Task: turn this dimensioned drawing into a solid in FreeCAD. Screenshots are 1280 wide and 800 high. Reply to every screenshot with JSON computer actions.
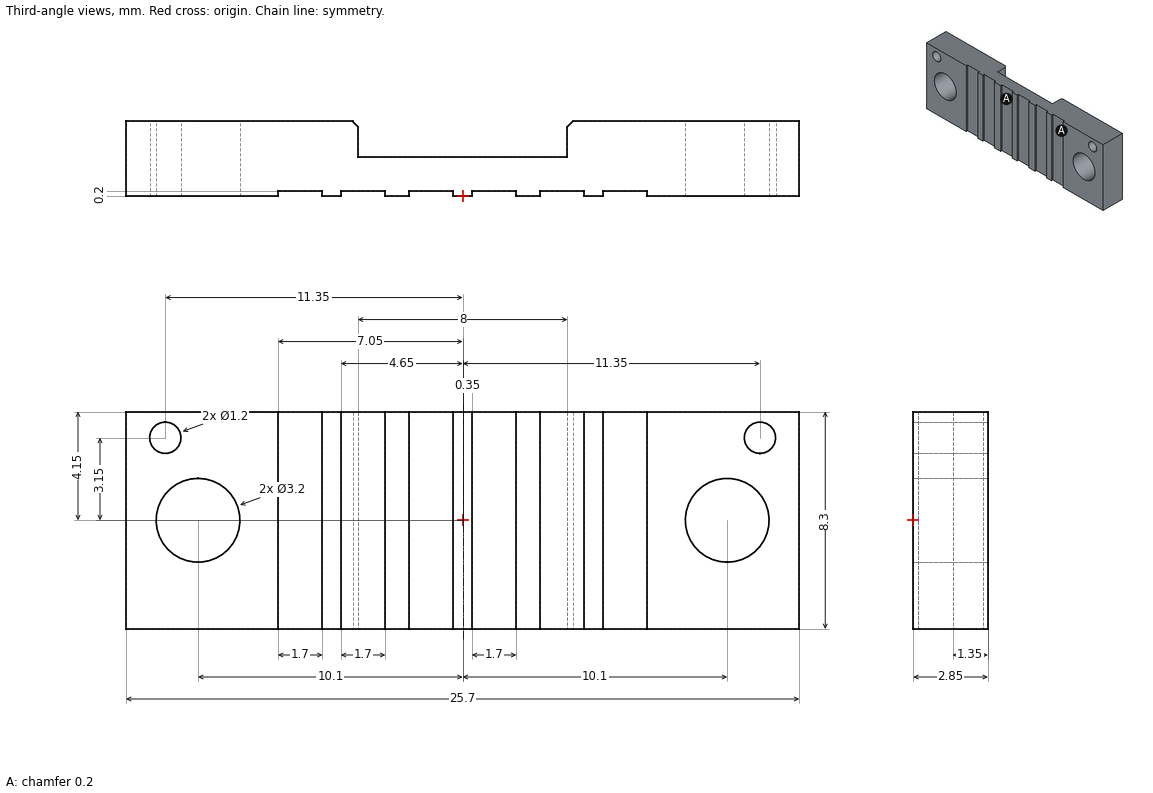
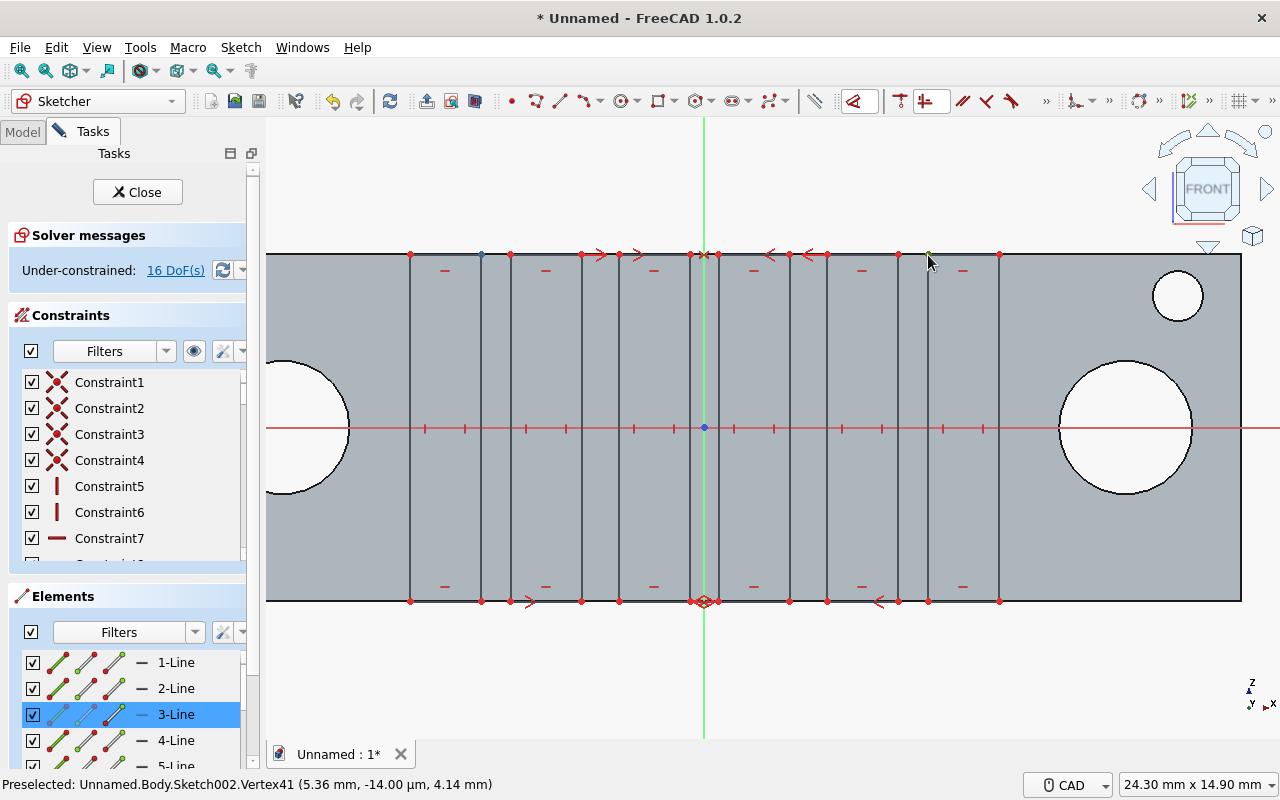
{"action": "left_click", "coordinate": [704, 671]}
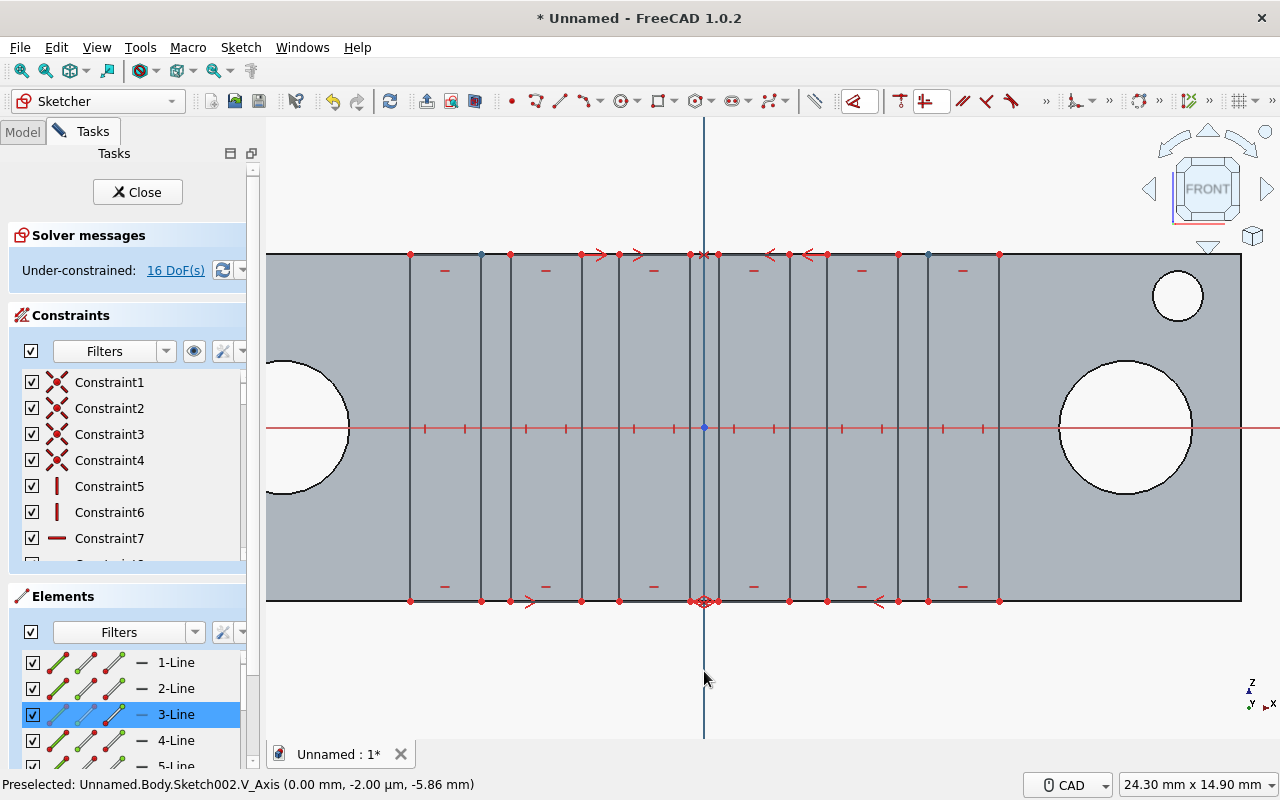
{"action": "key", "text": "s"}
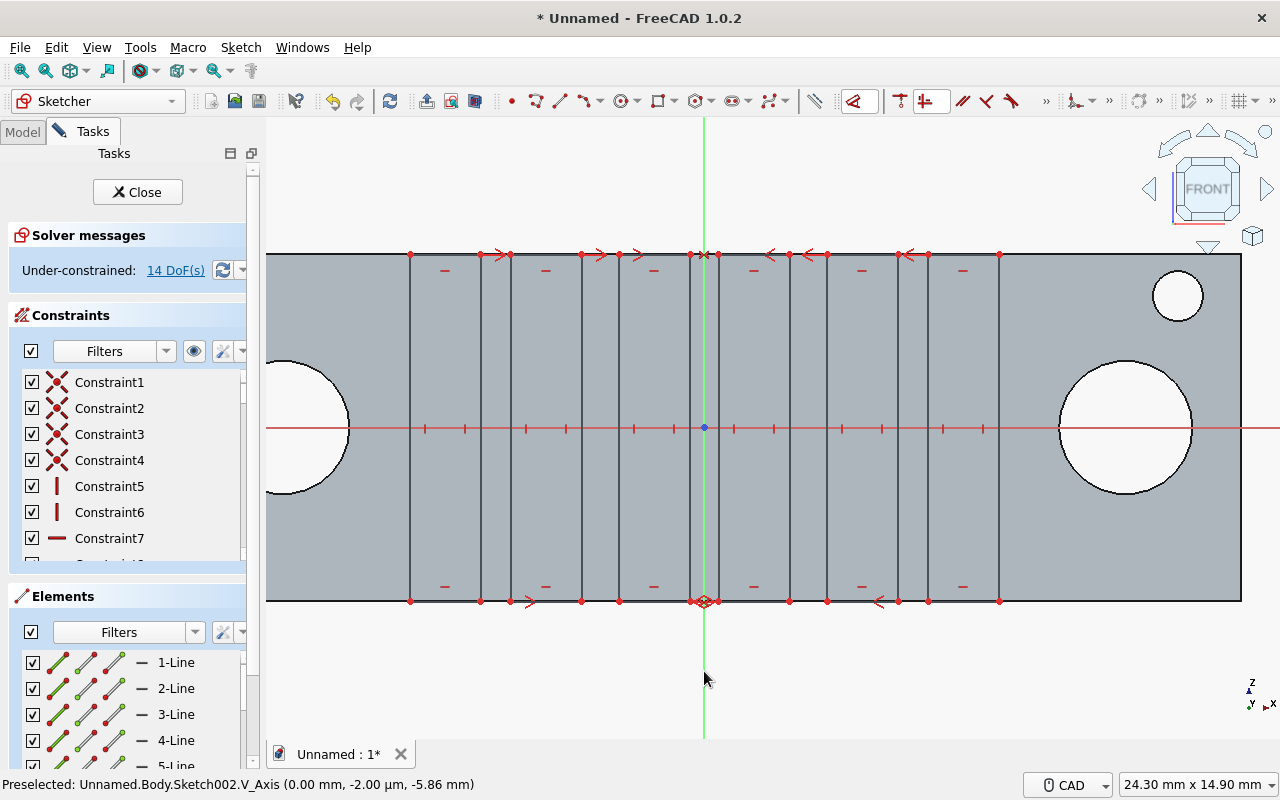
{"action": "left_click", "coordinate": [410, 602]}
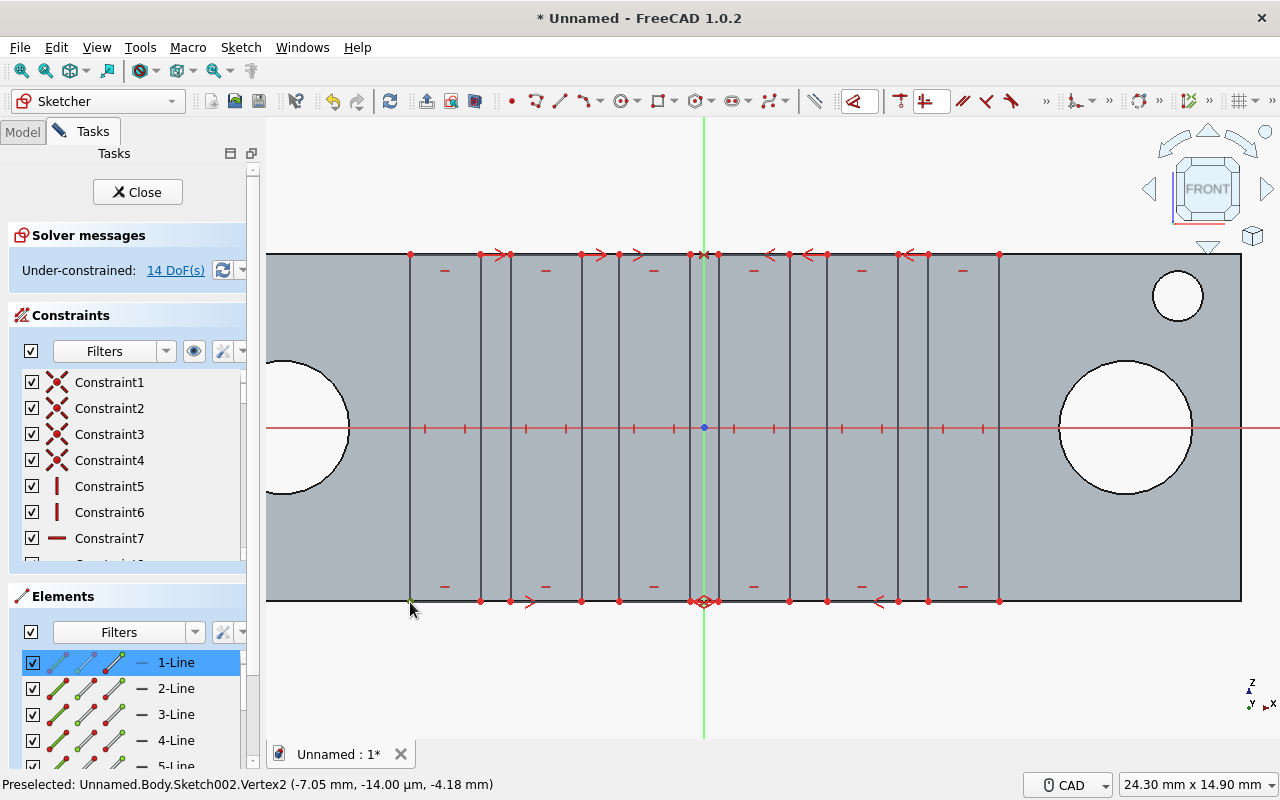
{"action": "left_click", "coordinate": [999, 602]}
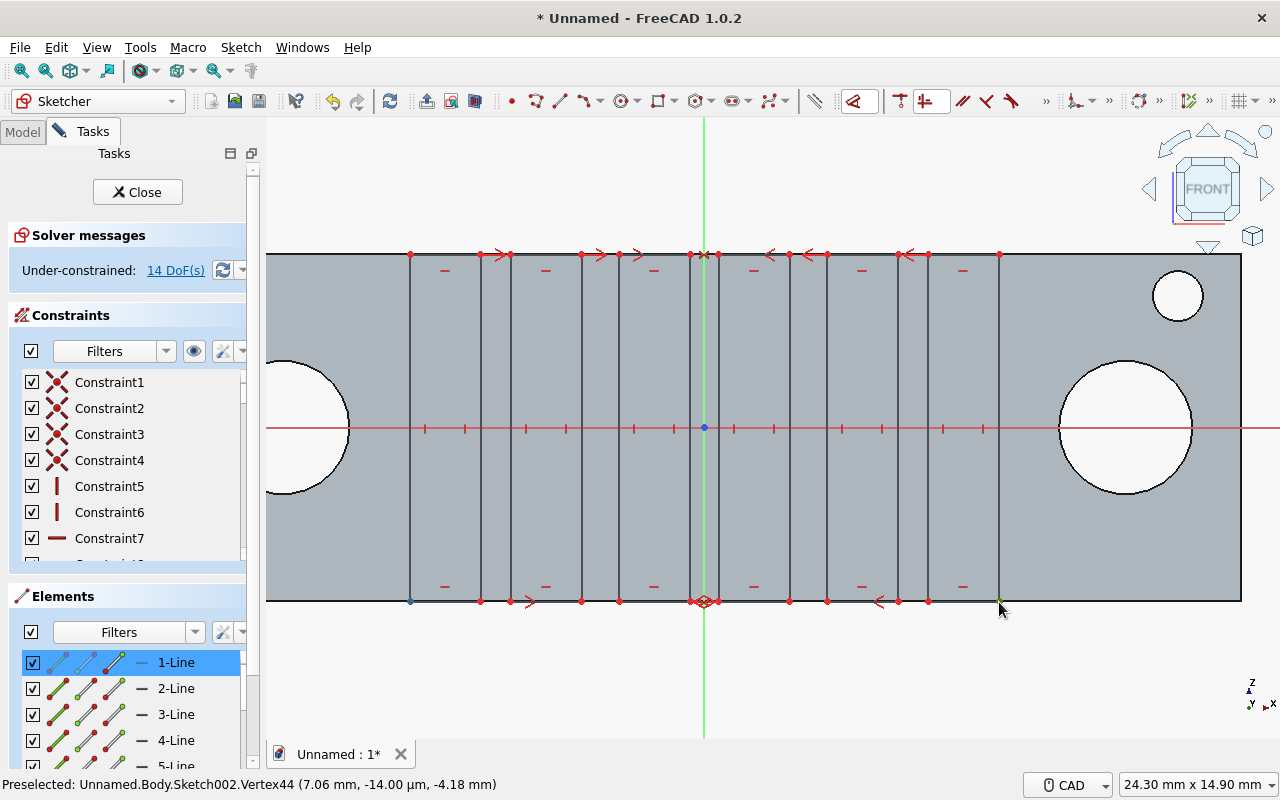
{"action": "left_click", "coordinate": [704, 671]}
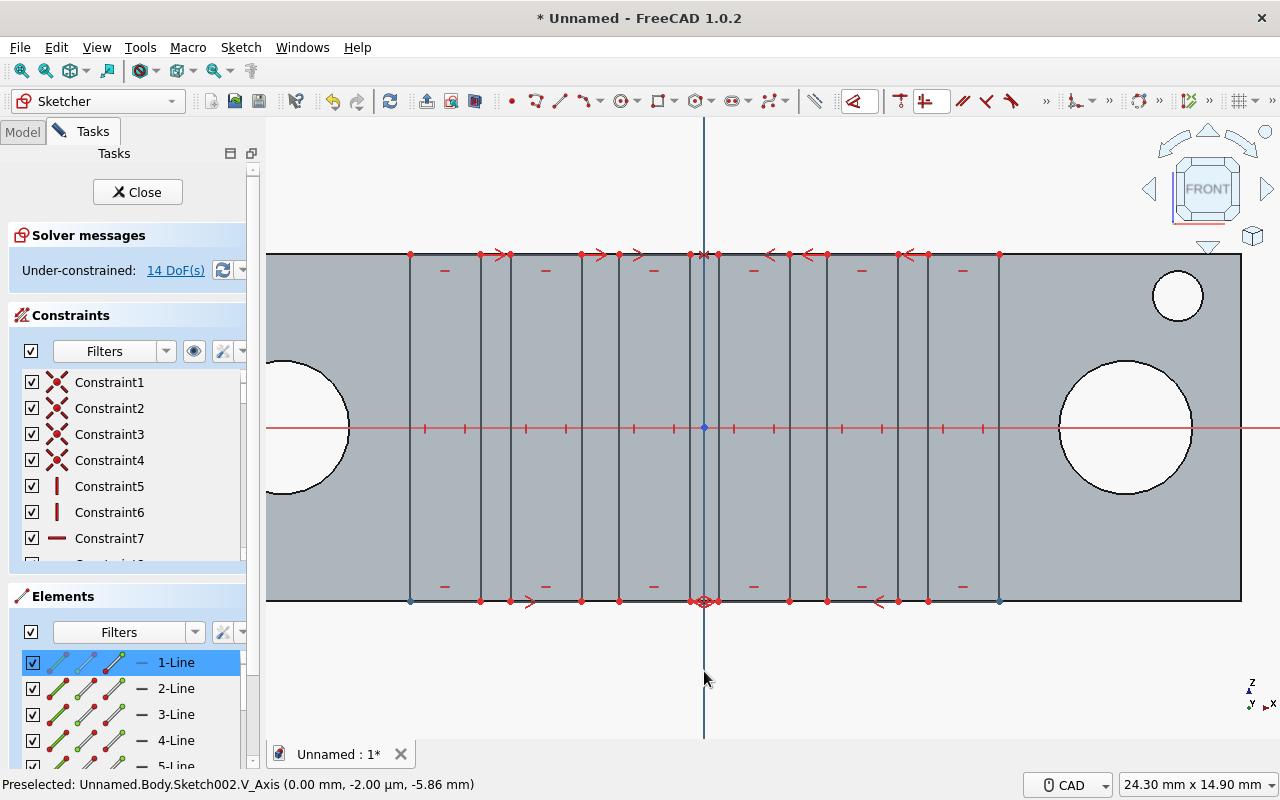
{"action": "key", "text": "s"}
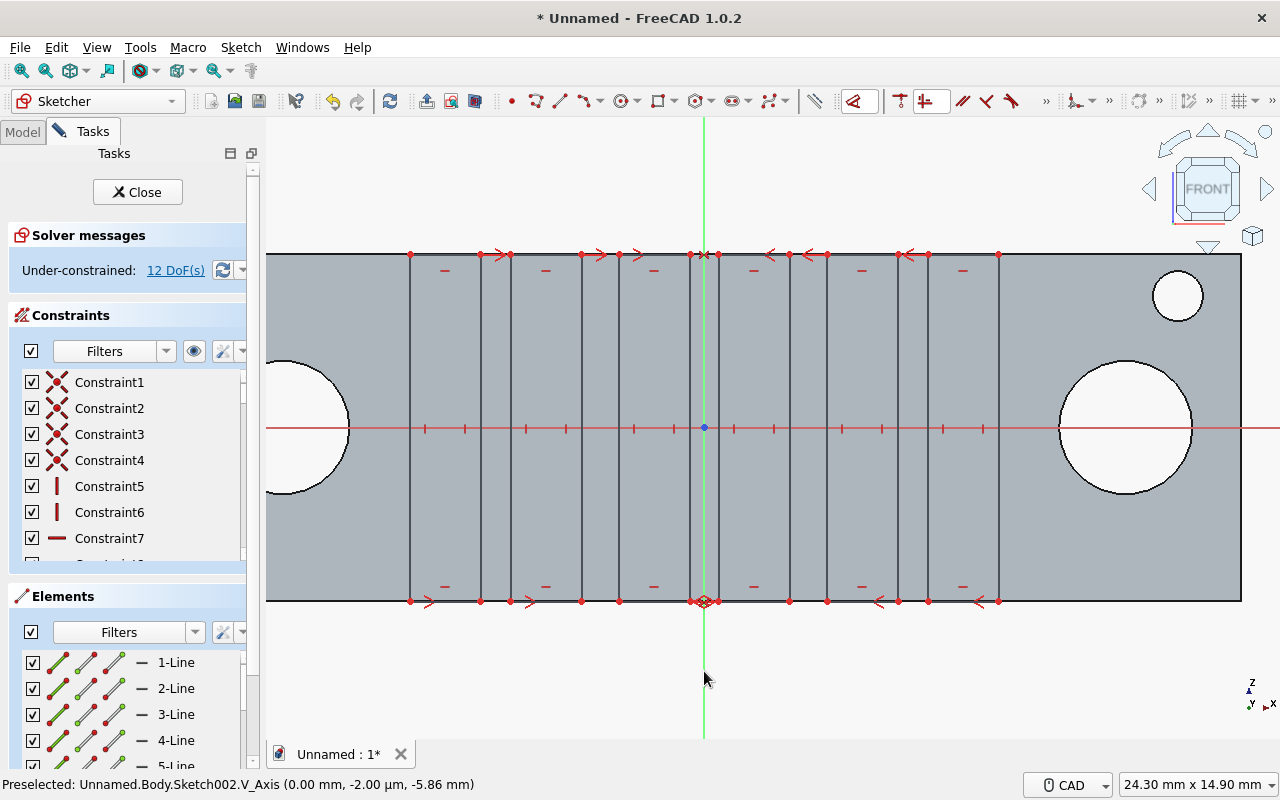
{"action": "key", "text": "d"}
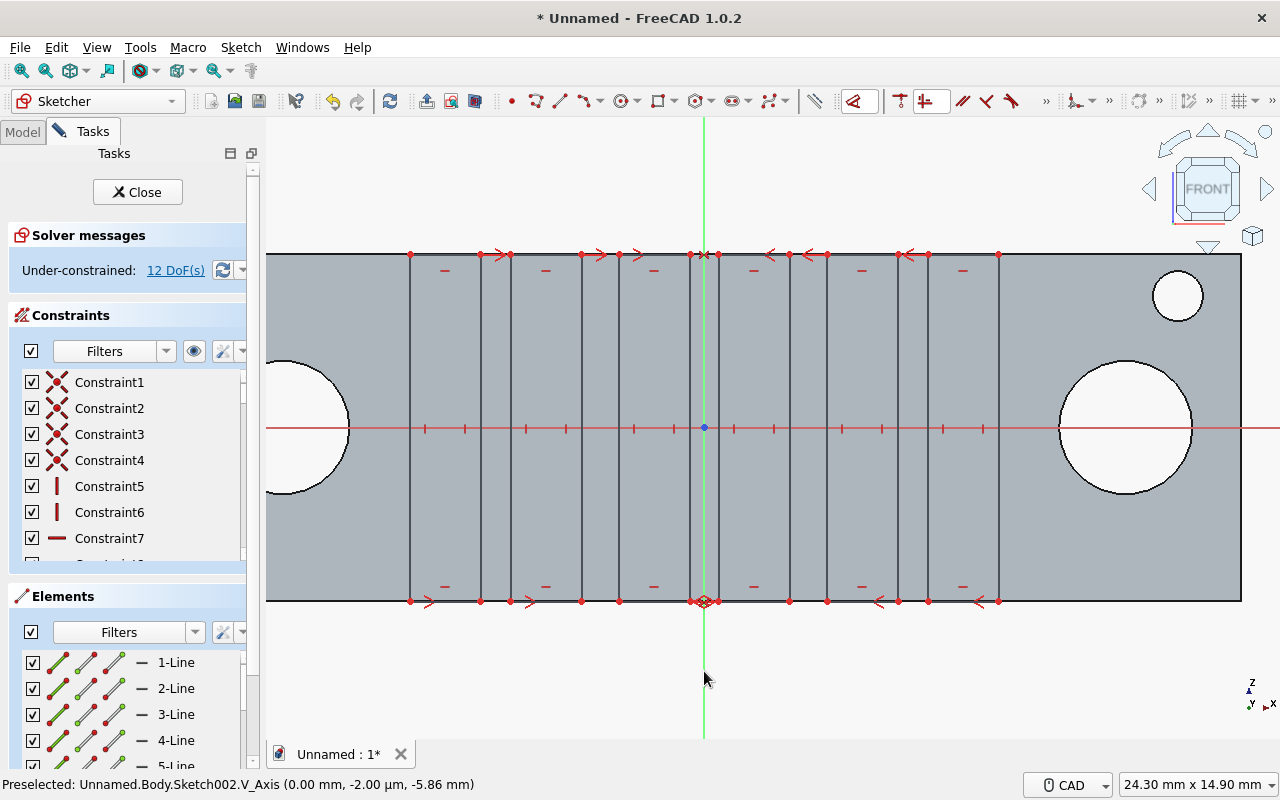
{"action": "left_click", "coordinate": [410, 359]}
{"action": "left_click", "coordinate": [376, 349]}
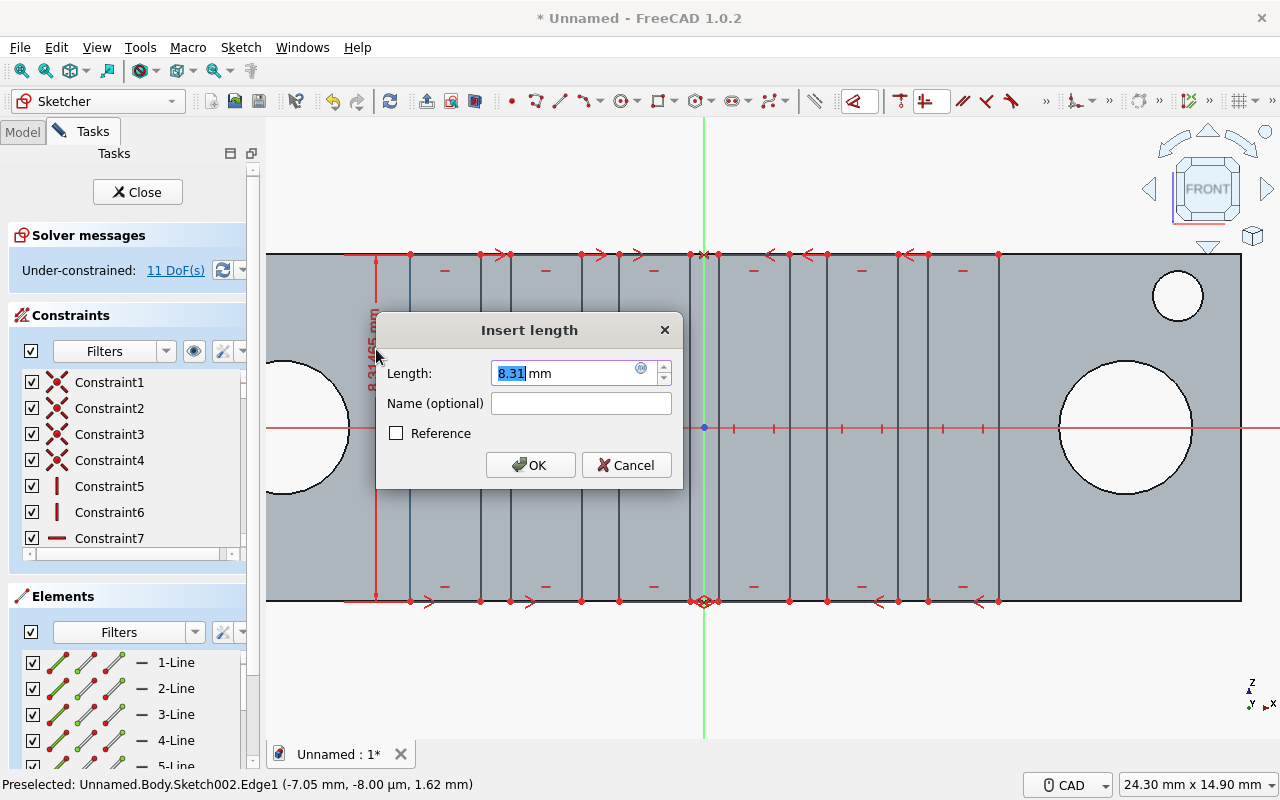
{"action": "type", "text": "8.3"}
{"action": "key", "text": "Return"}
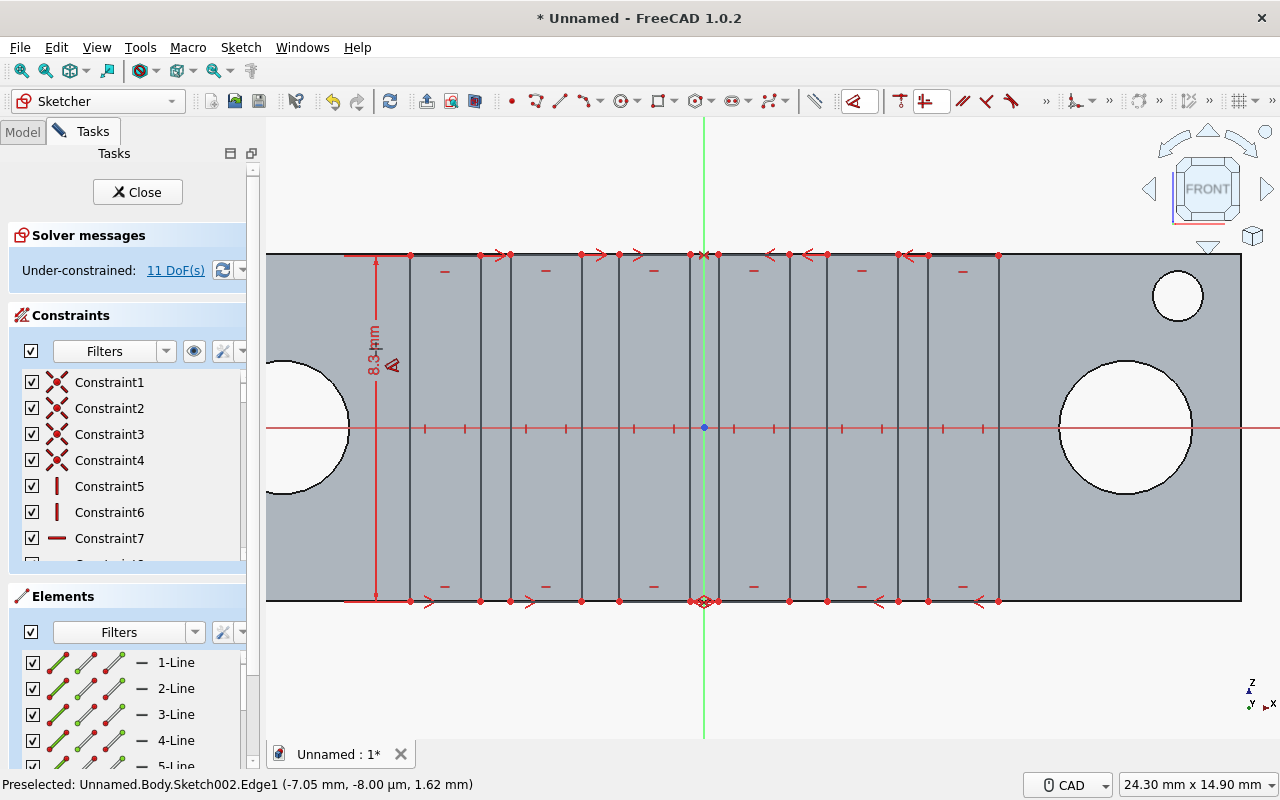
{"action": "left_click", "coordinate": [431, 602]}
{"action": "left_click", "coordinate": [445, 636]}